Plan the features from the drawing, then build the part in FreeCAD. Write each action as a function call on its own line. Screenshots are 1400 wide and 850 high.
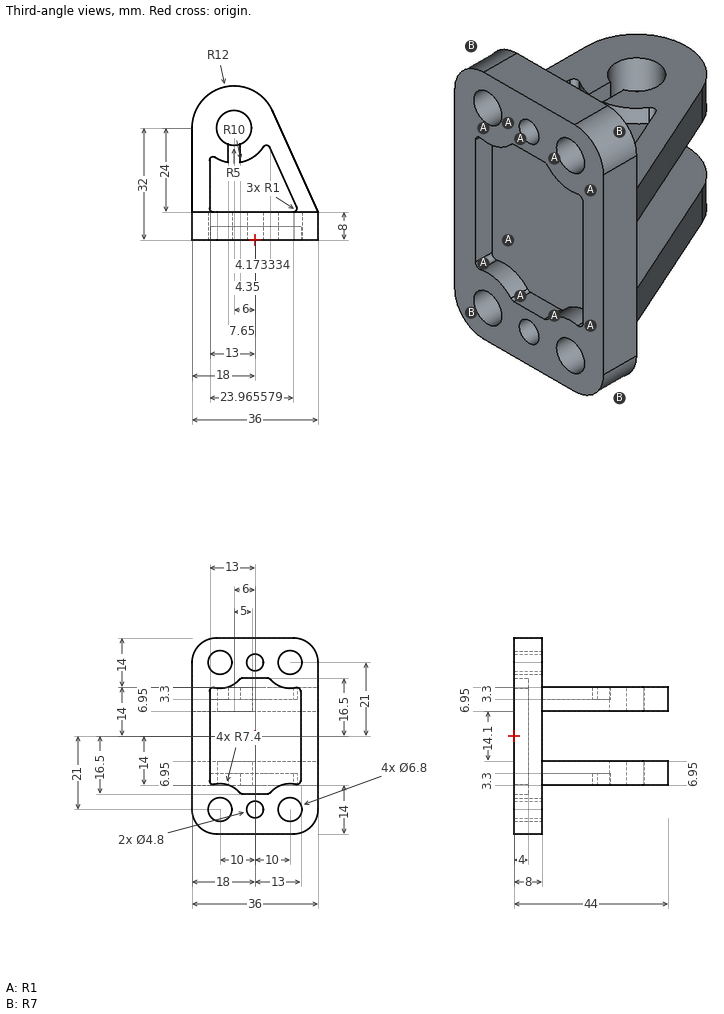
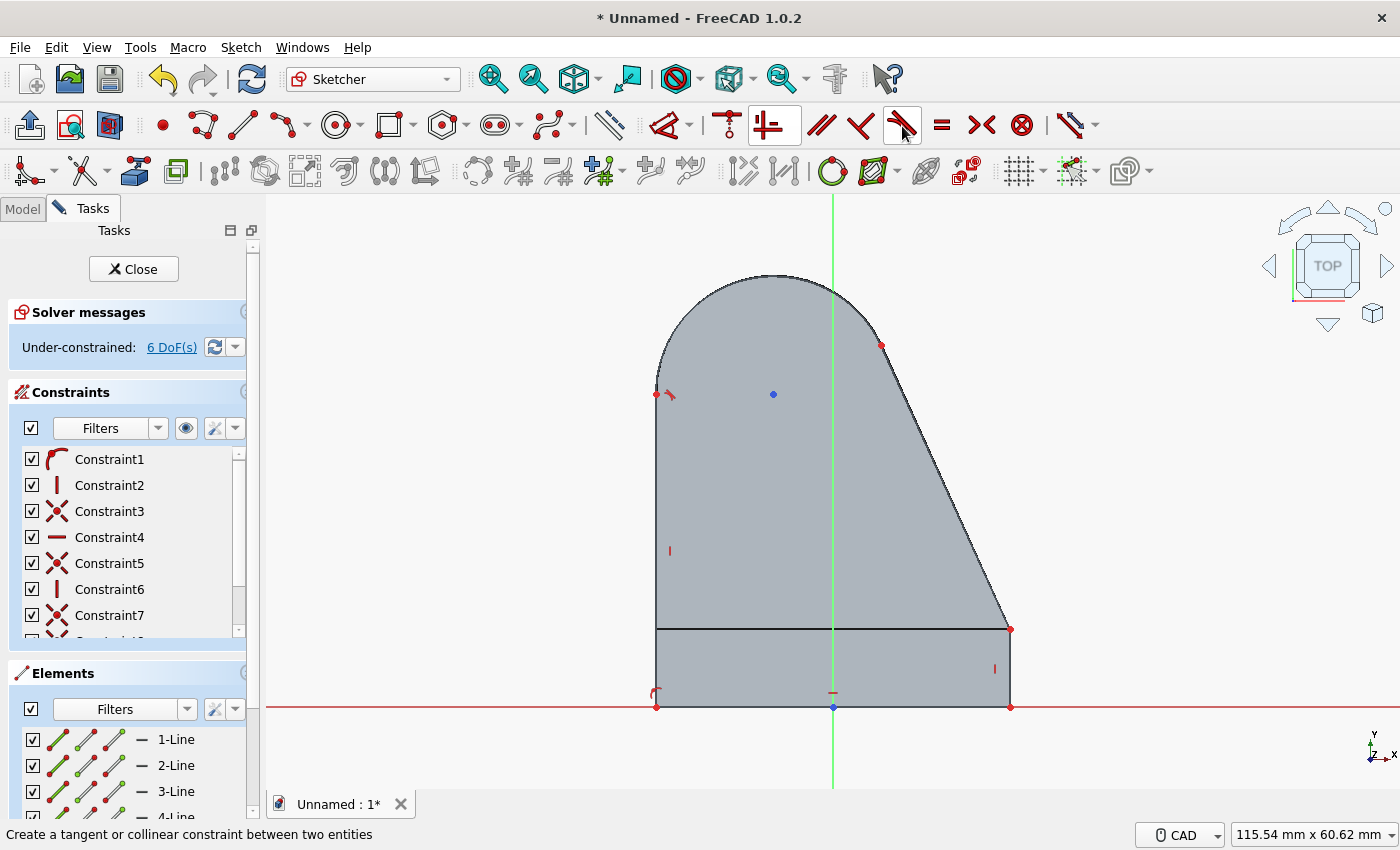
click(971, 545)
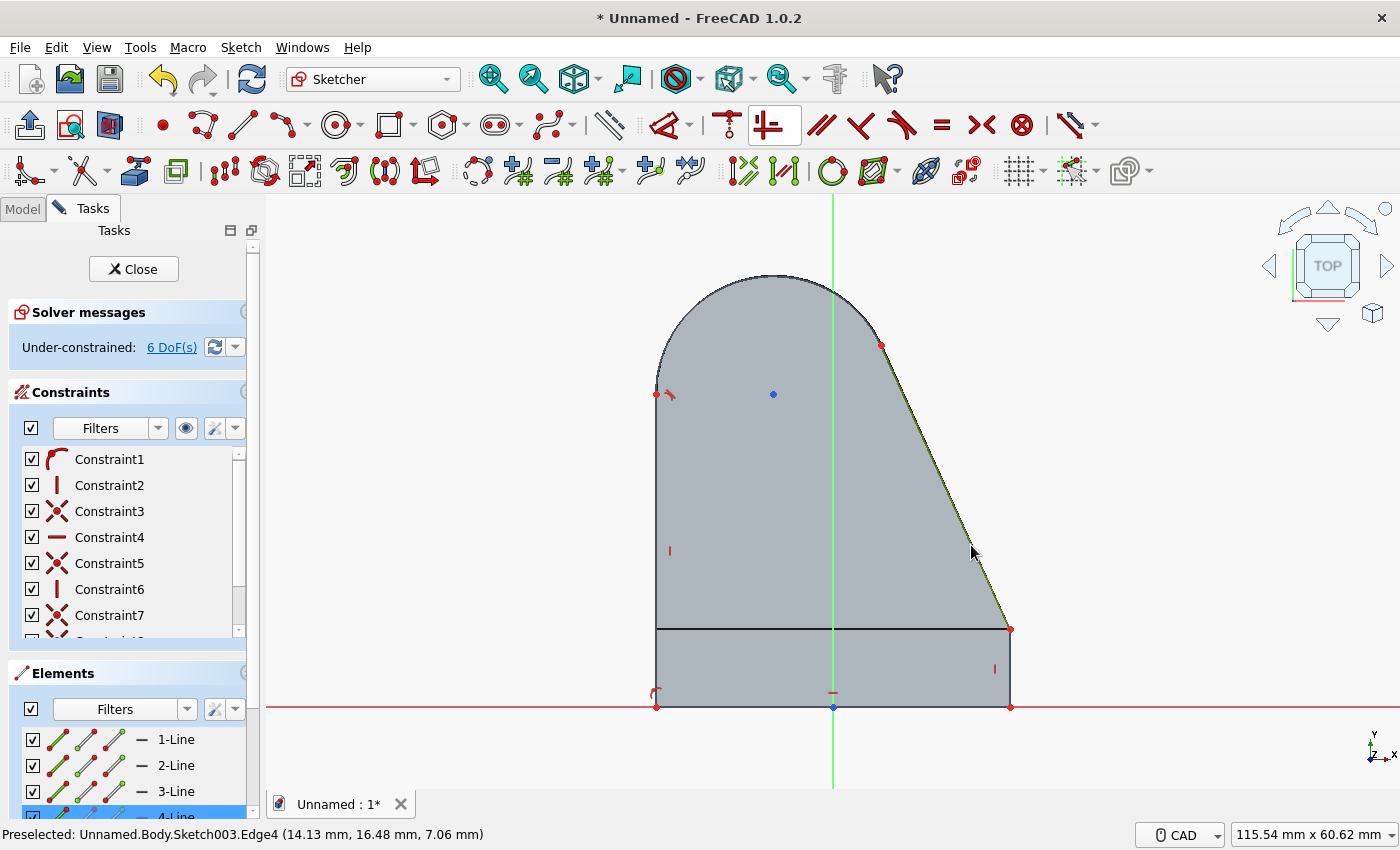
click(812, 283)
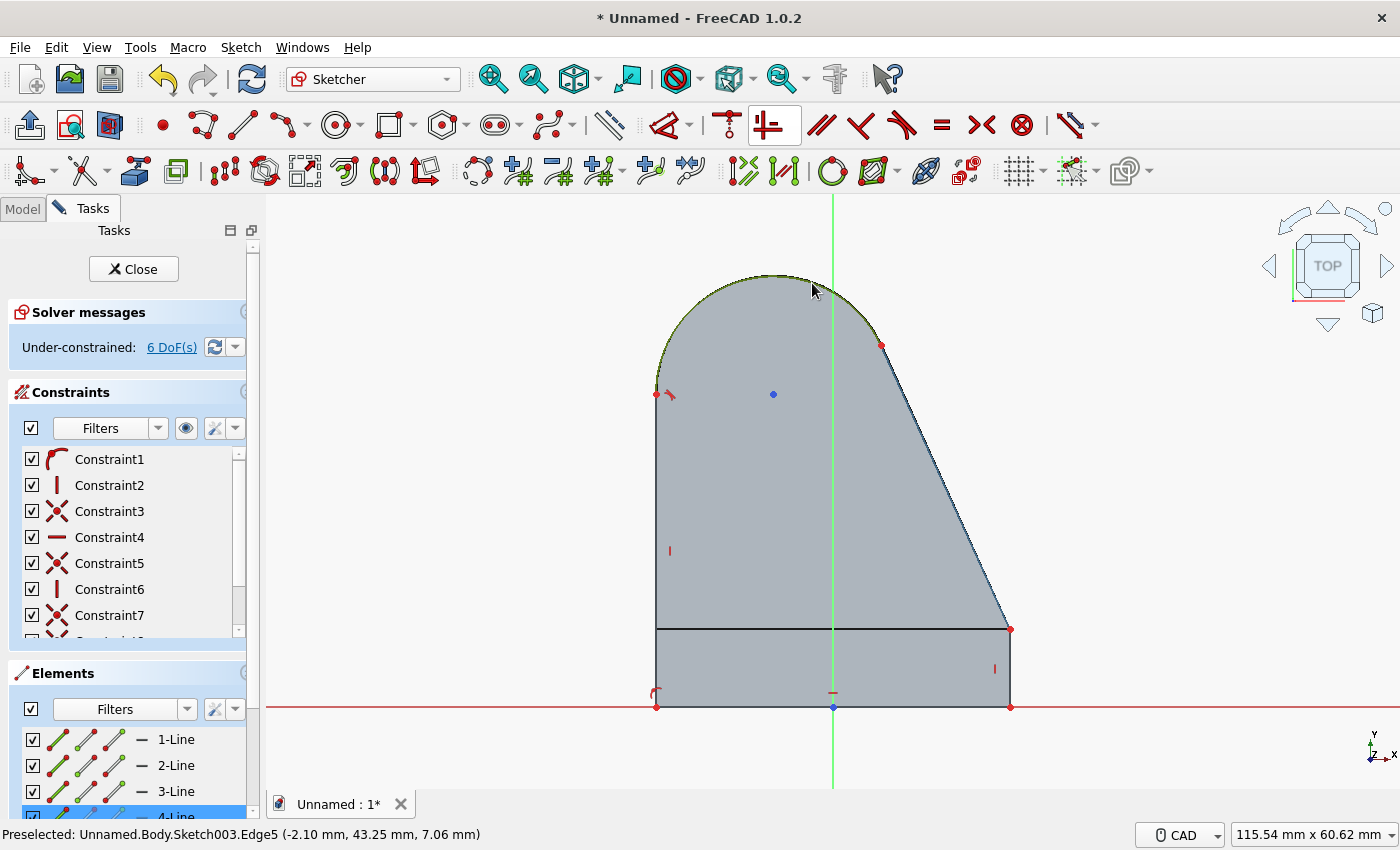
key(t)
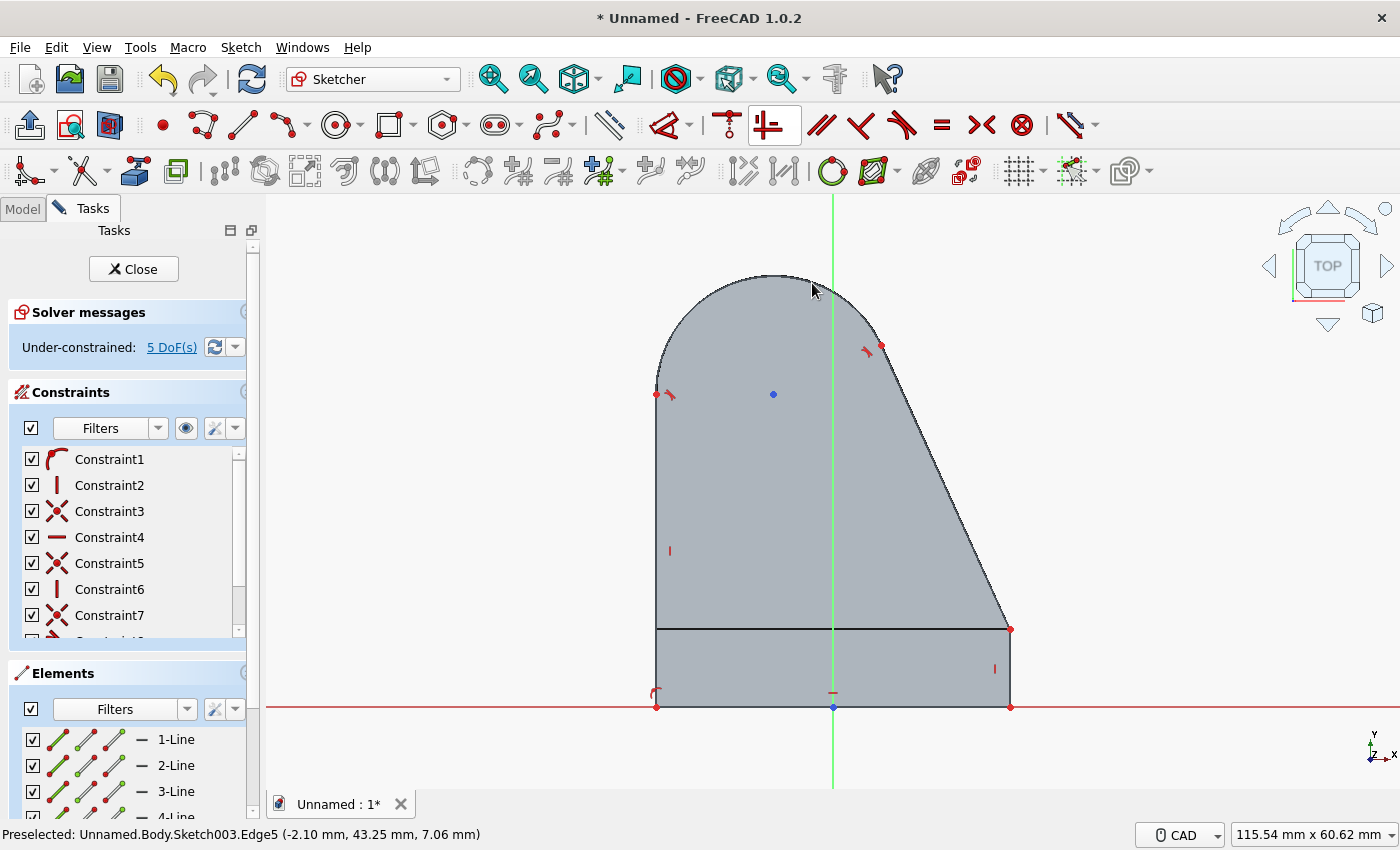
click(812, 283)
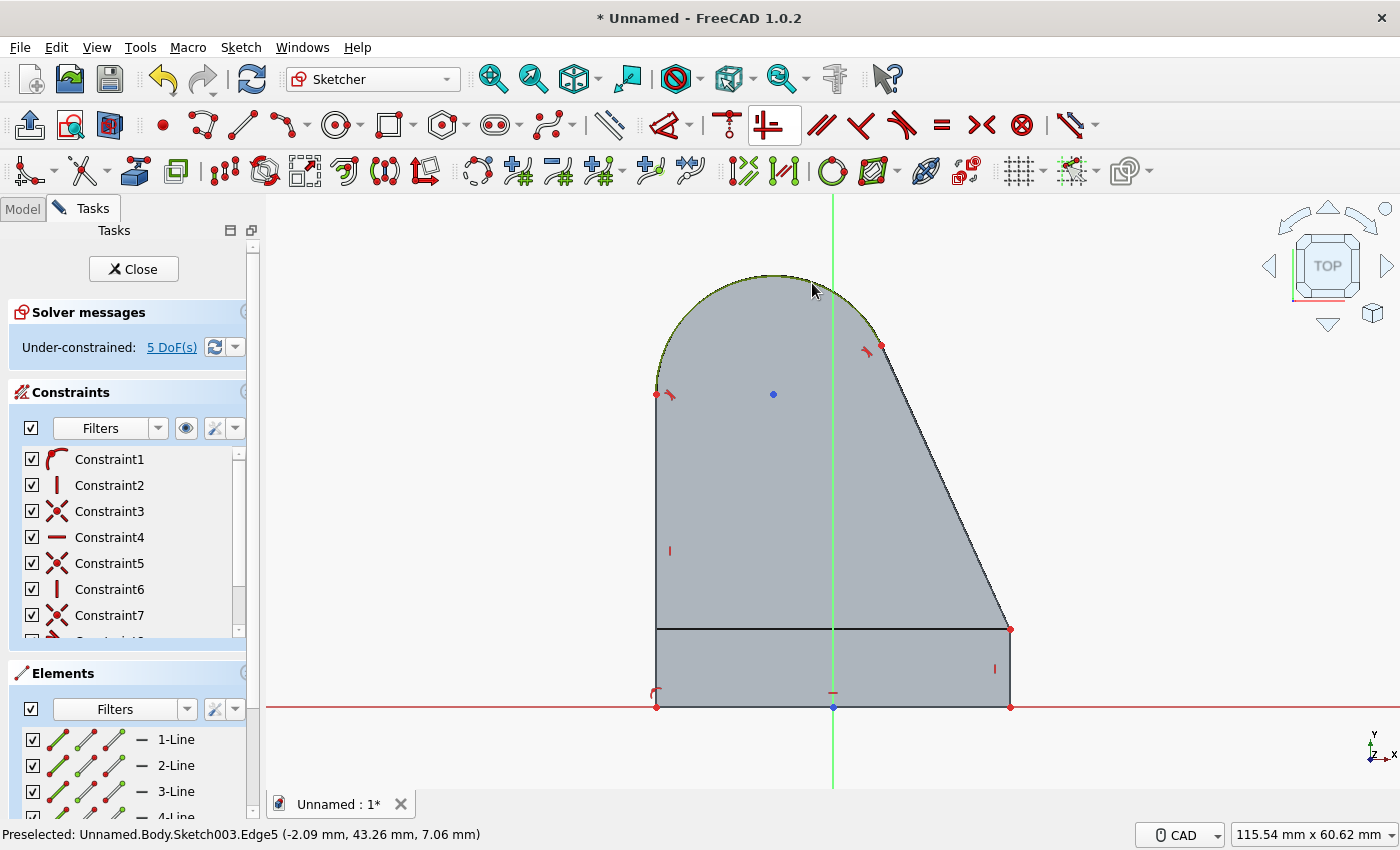
key(k)
key(r)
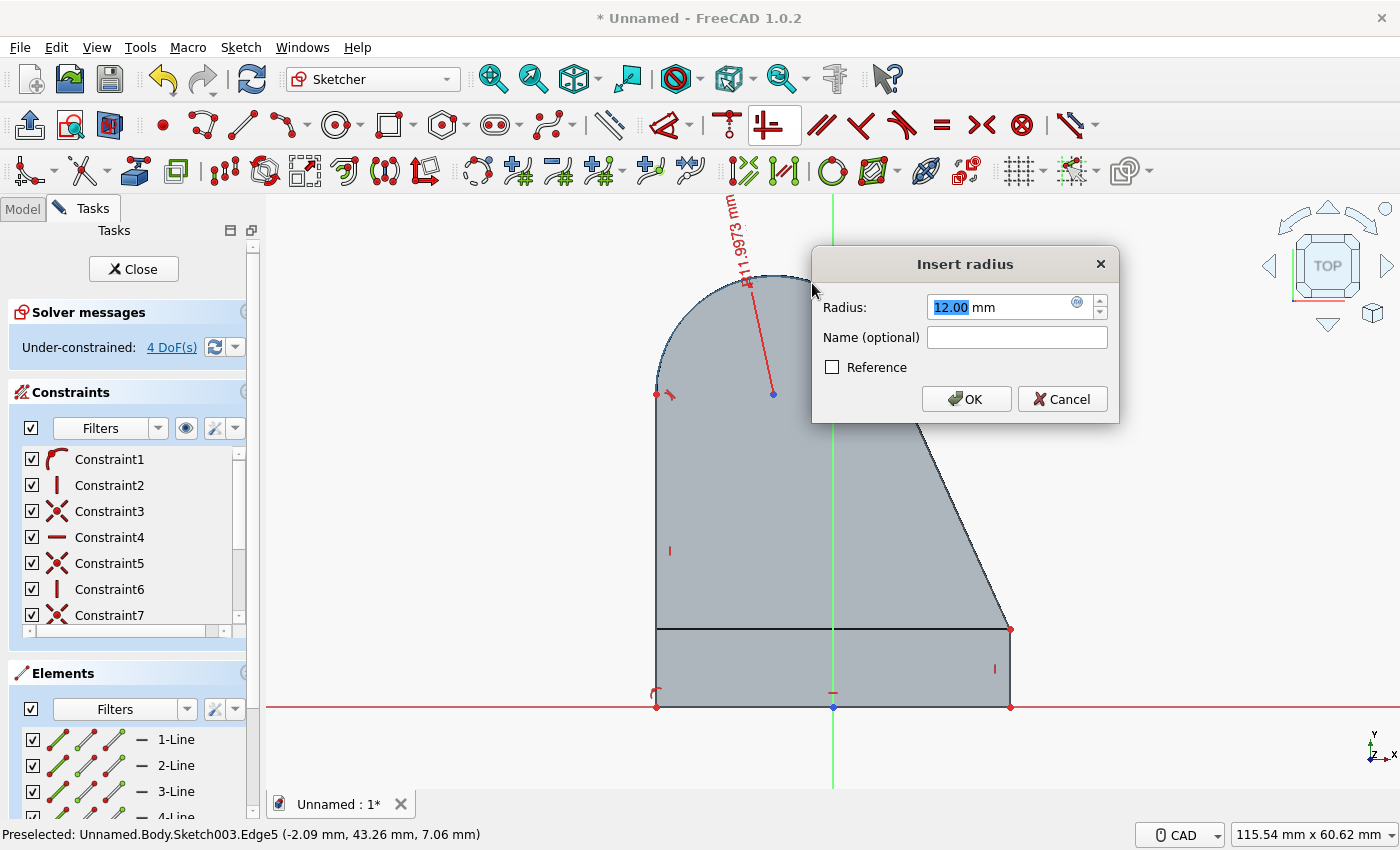
text(12)
key(Return)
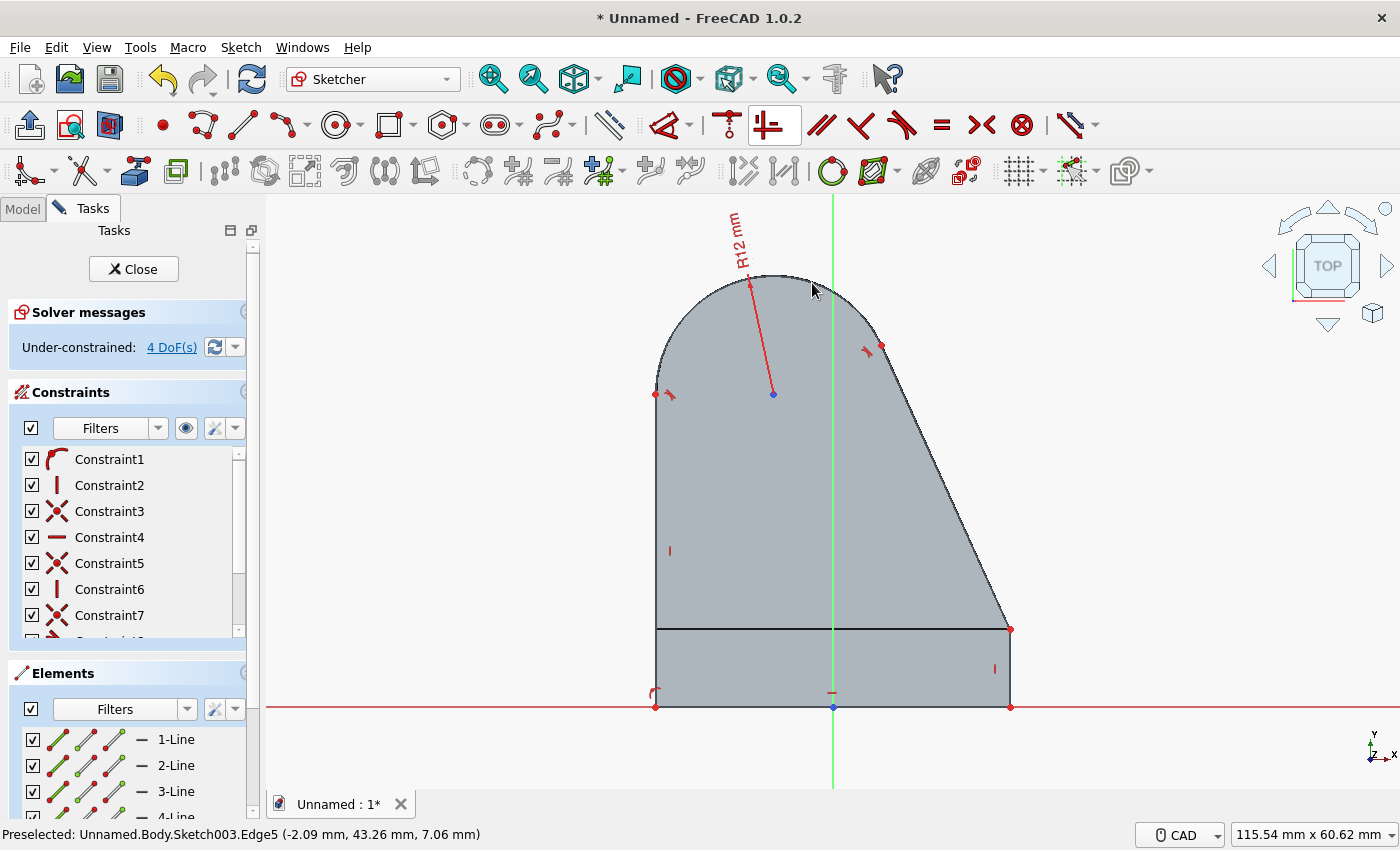
click(1010, 684)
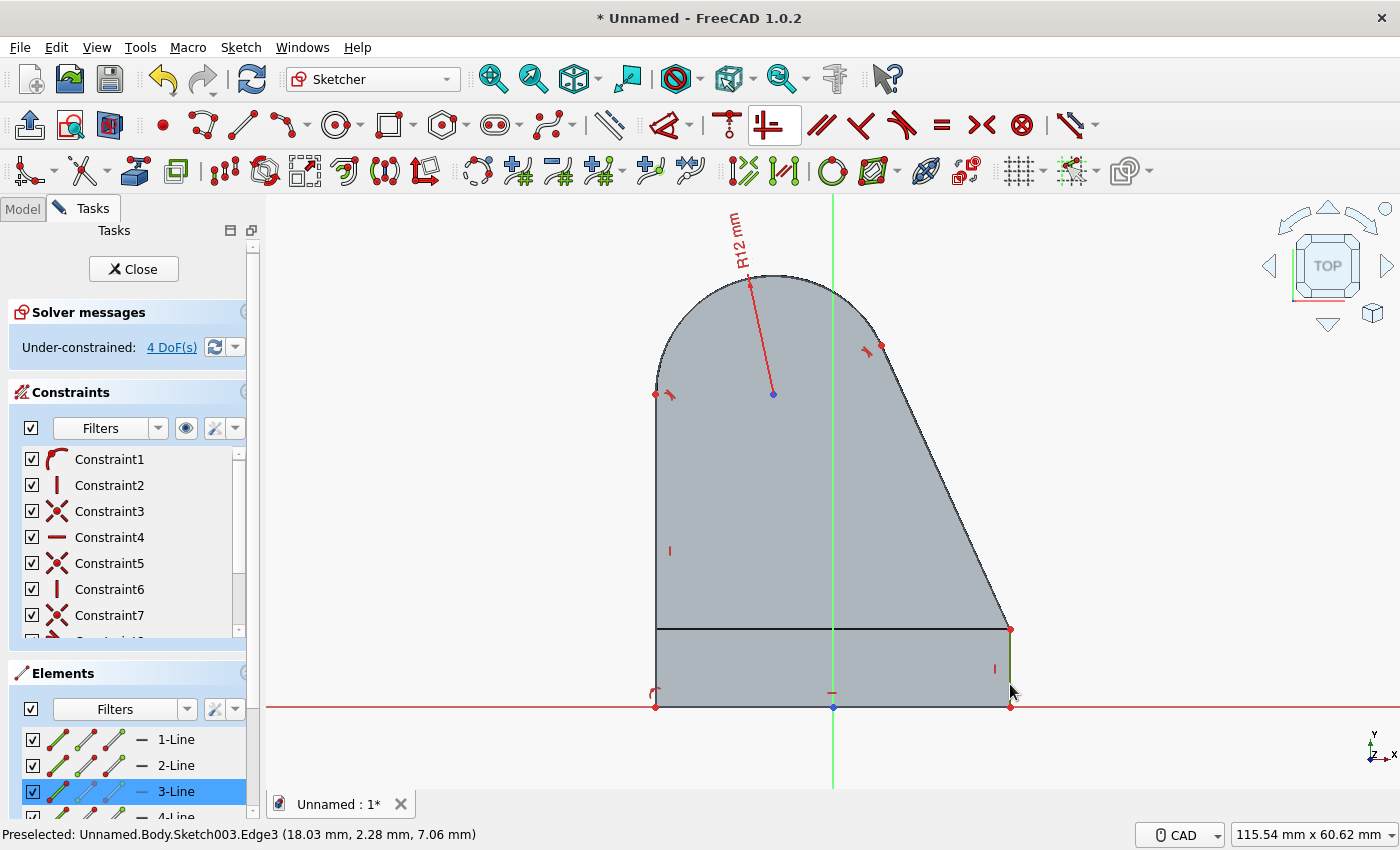
key(i)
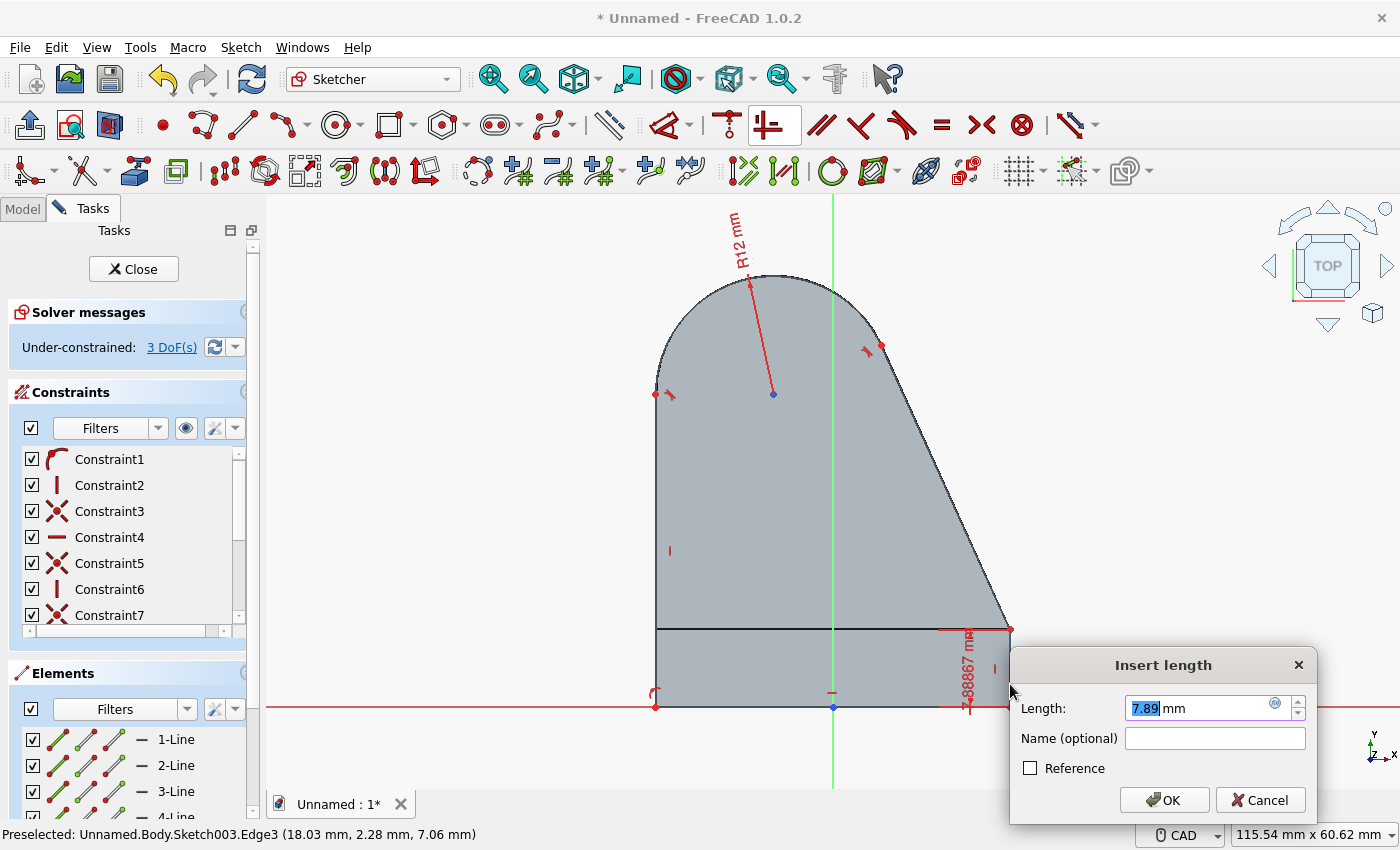
text(8)
key(Return)